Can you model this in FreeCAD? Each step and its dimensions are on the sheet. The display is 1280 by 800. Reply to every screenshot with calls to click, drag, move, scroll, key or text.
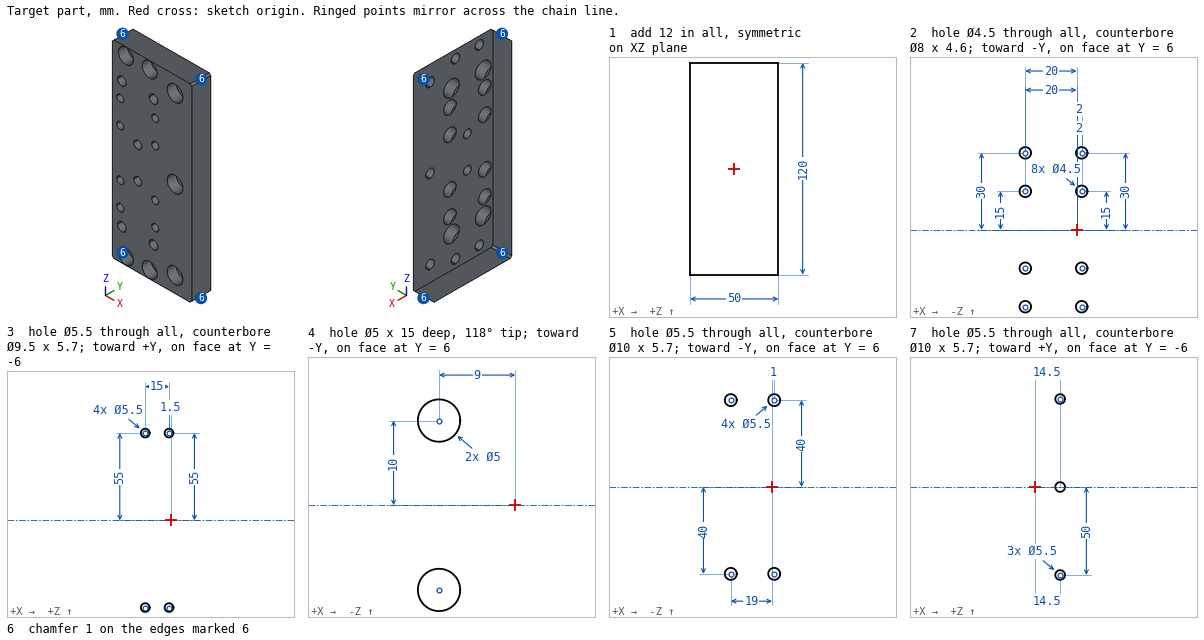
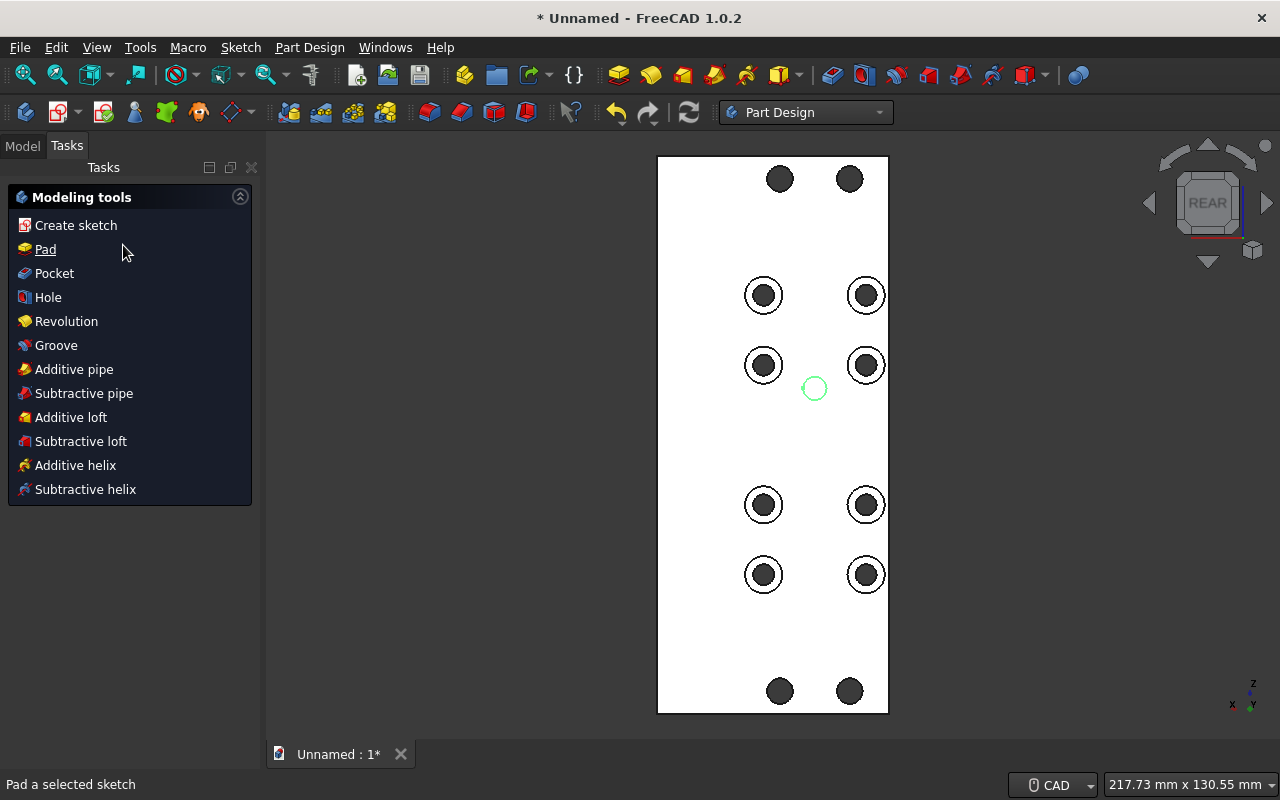
click(866, 76)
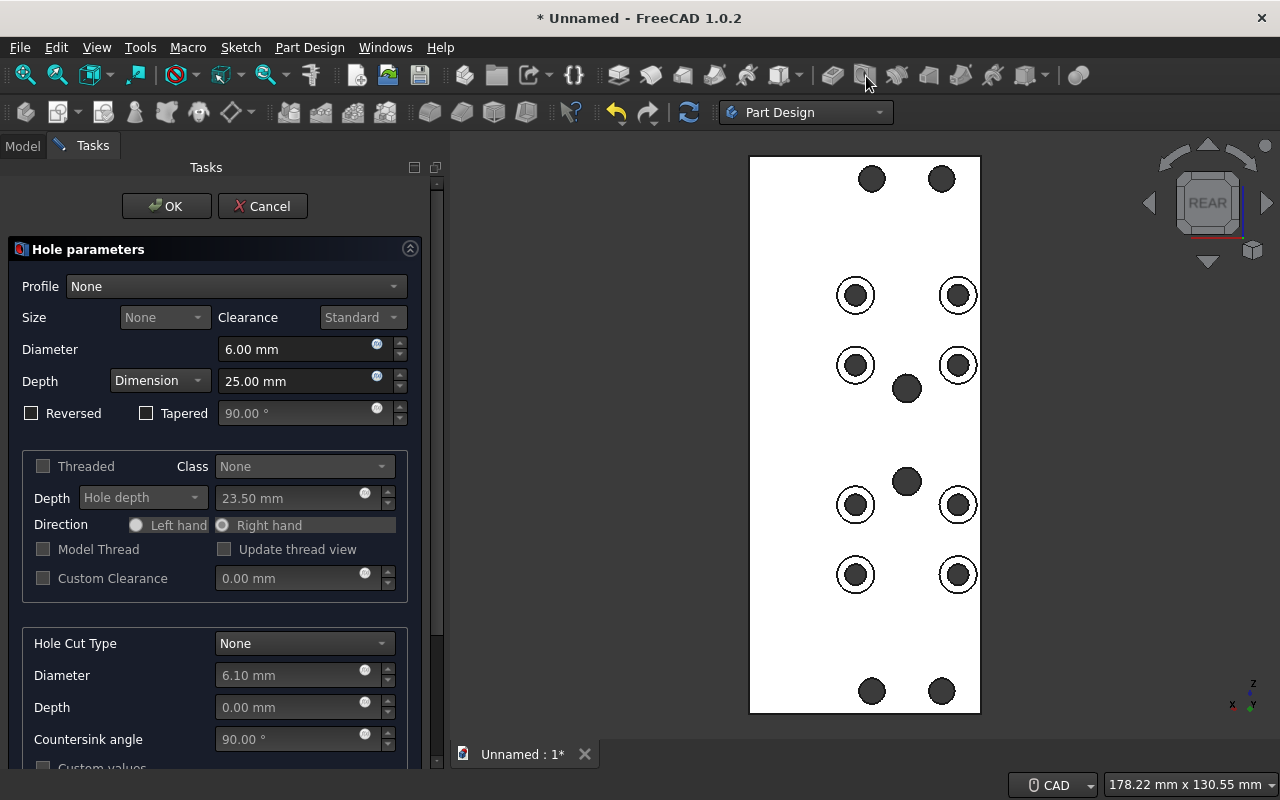
triple_click(305, 349)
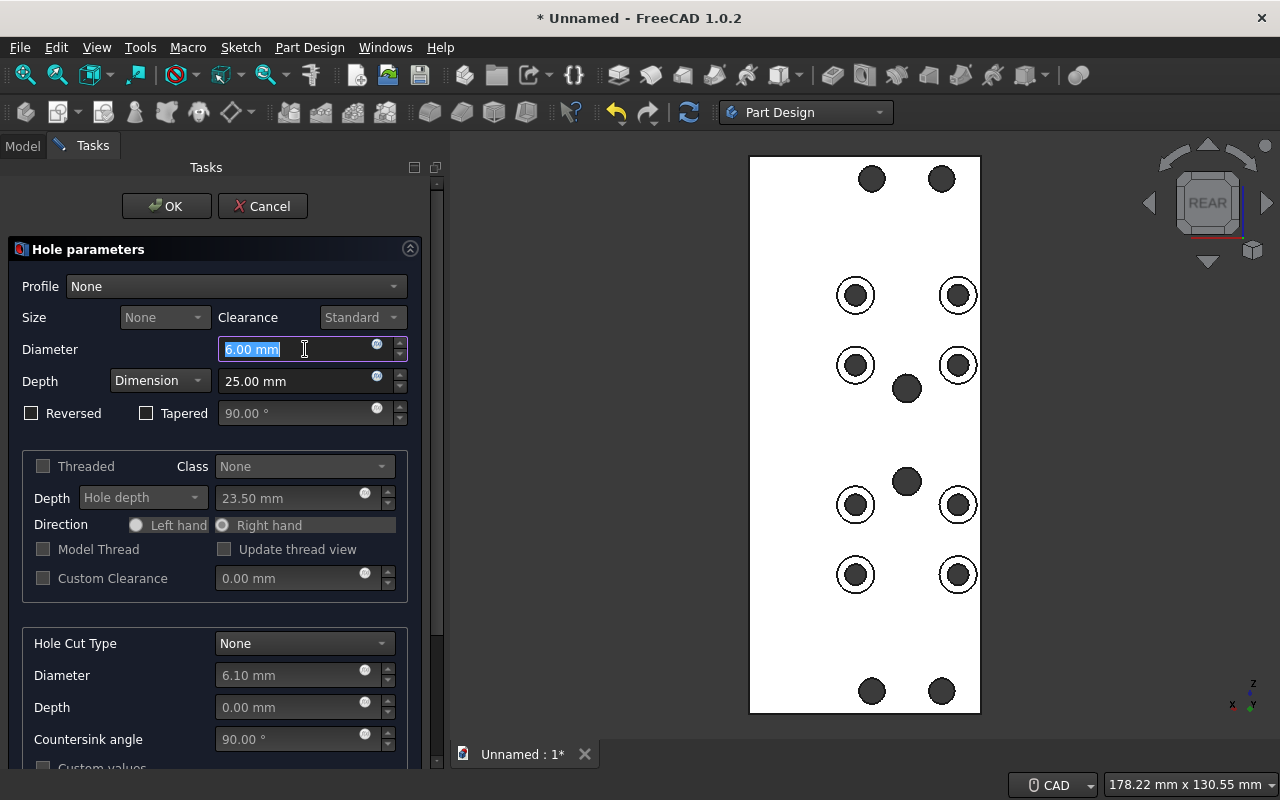
text(5)
key(Tab)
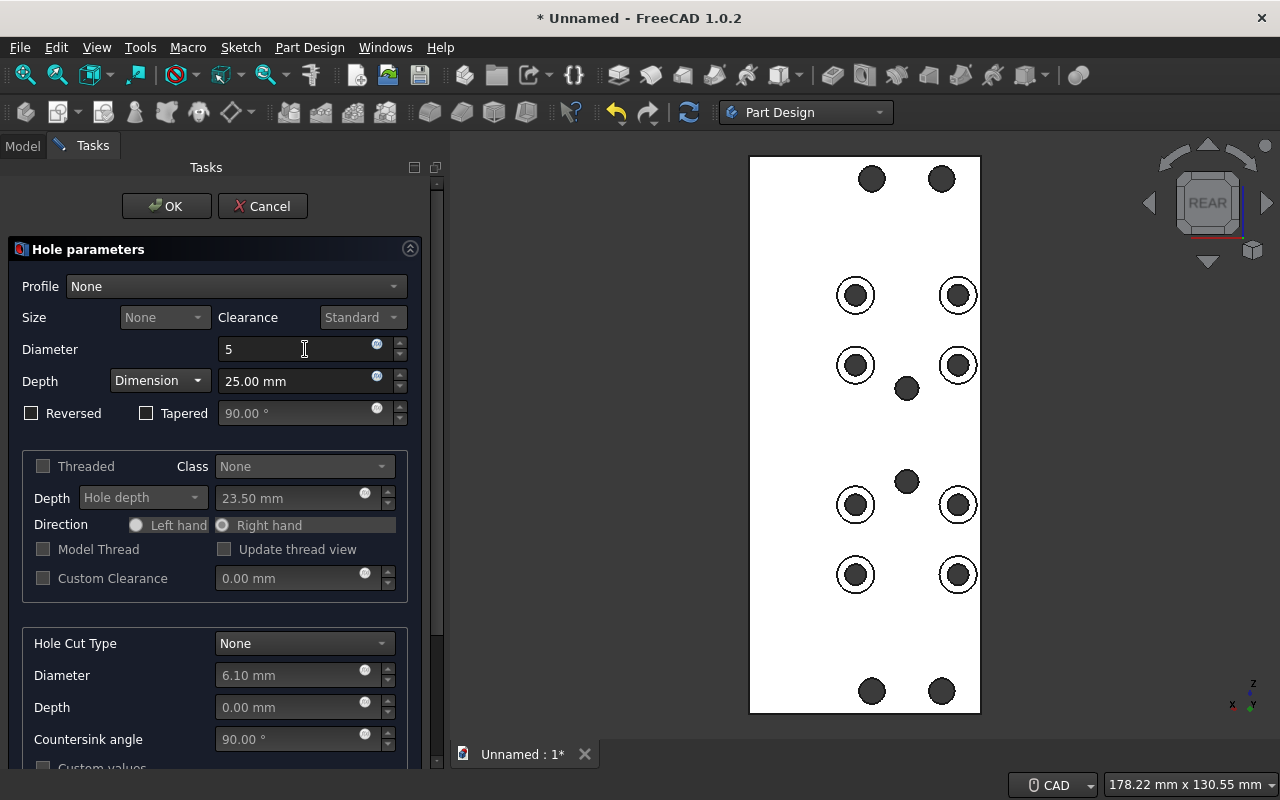
triple_click(305, 381)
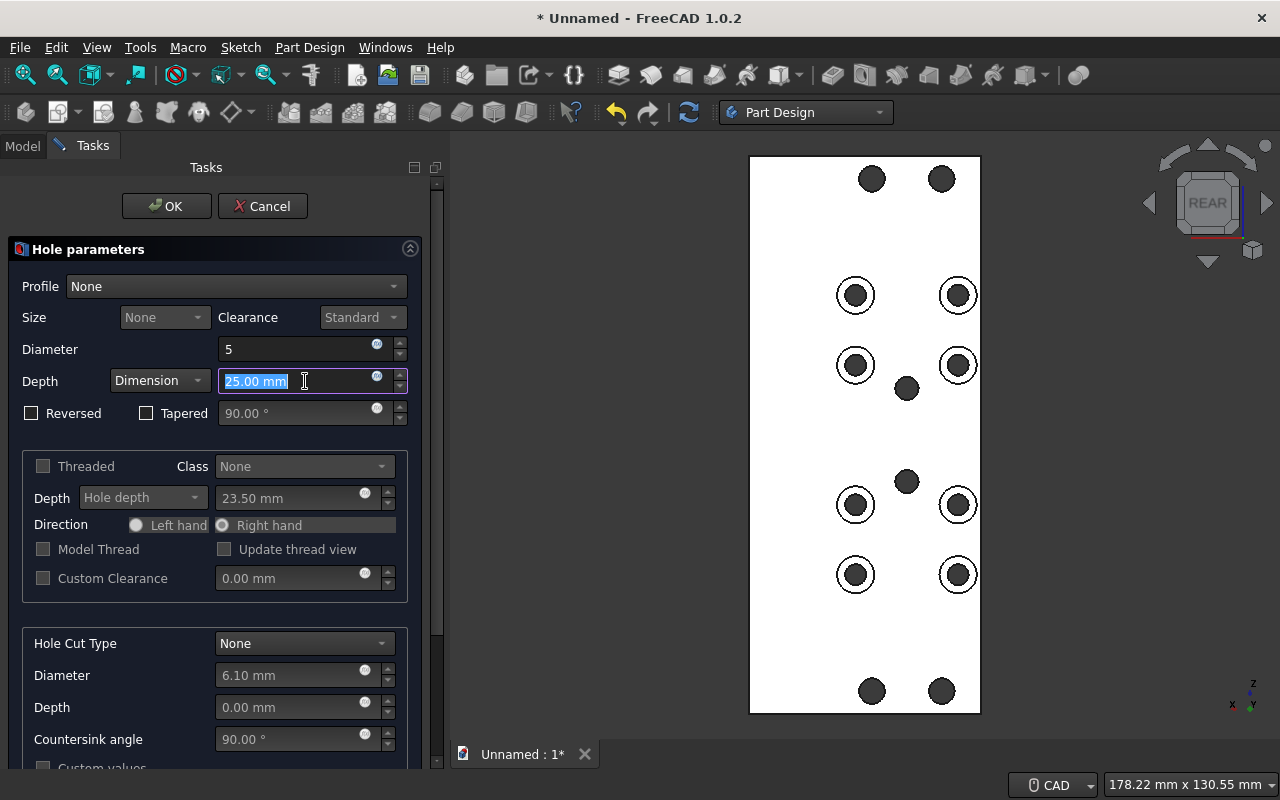
text(15)
key(Tab)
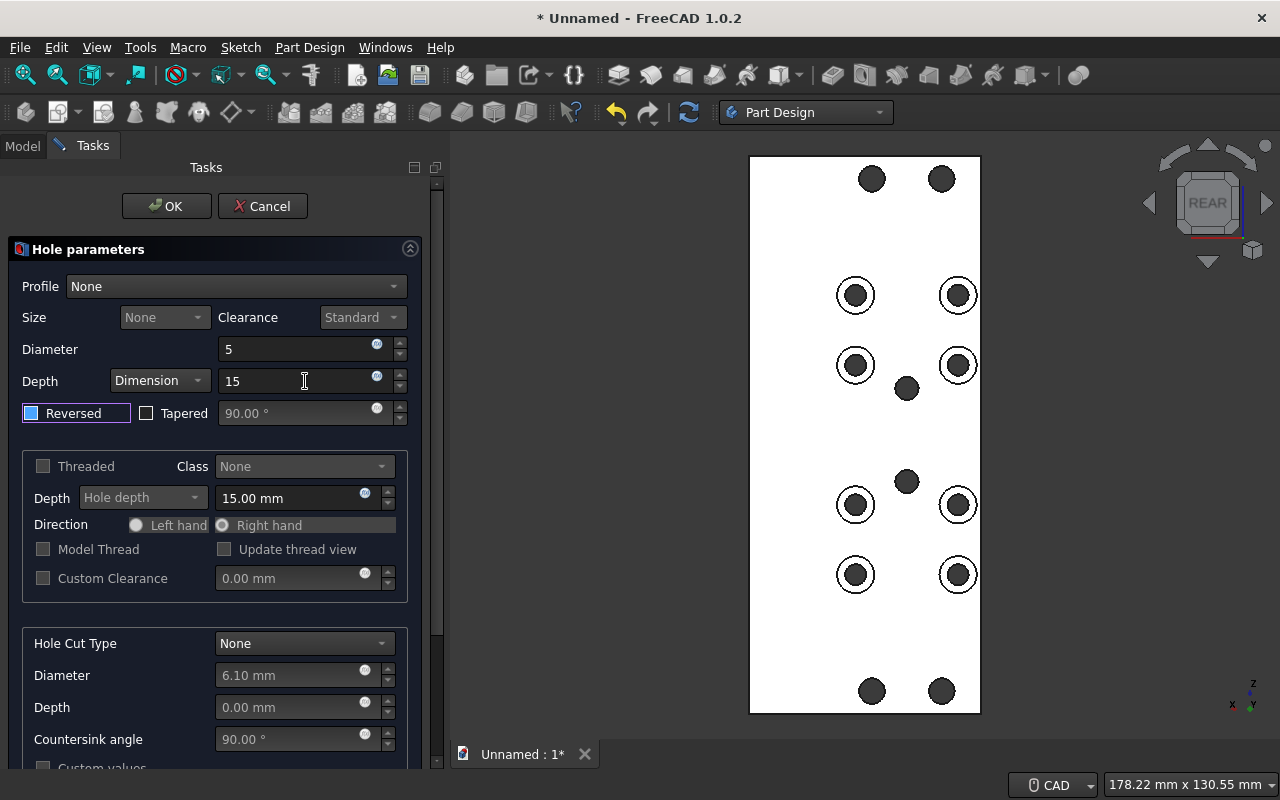
click(167, 206)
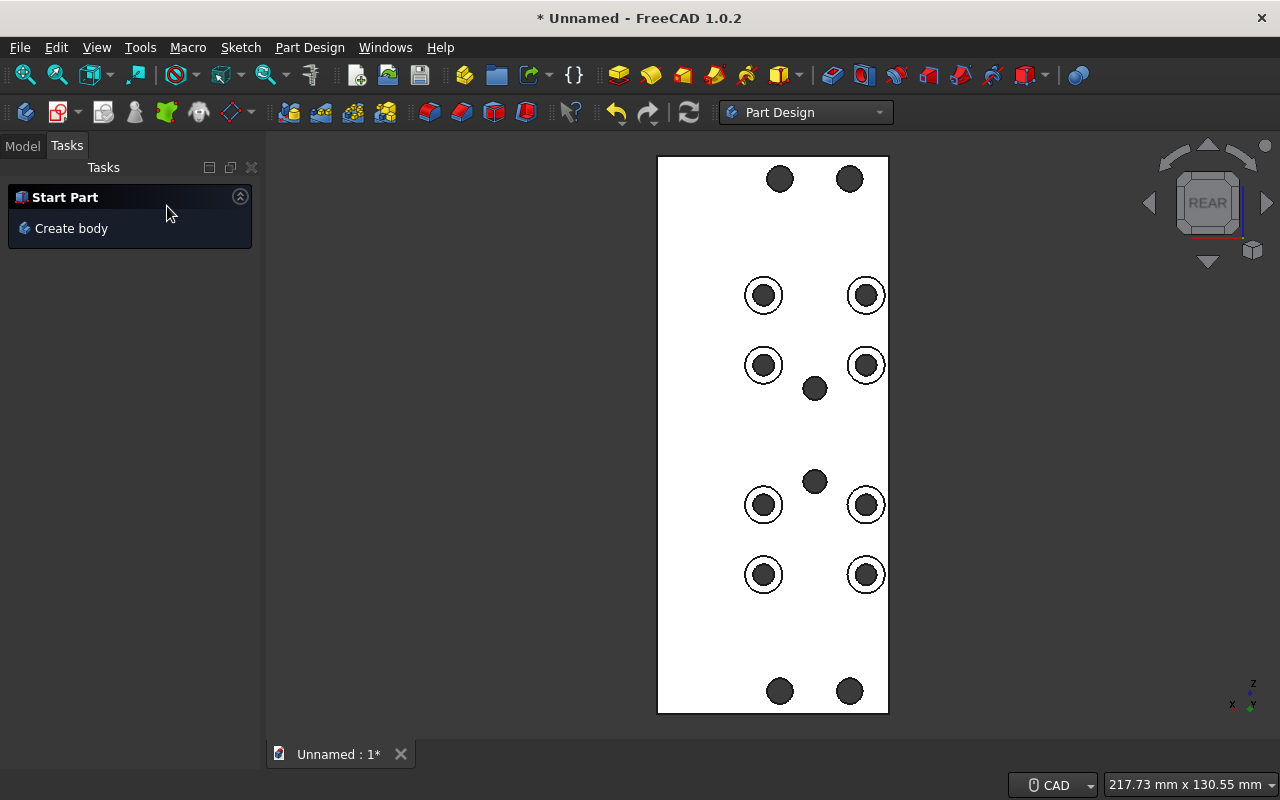
click(740, 434)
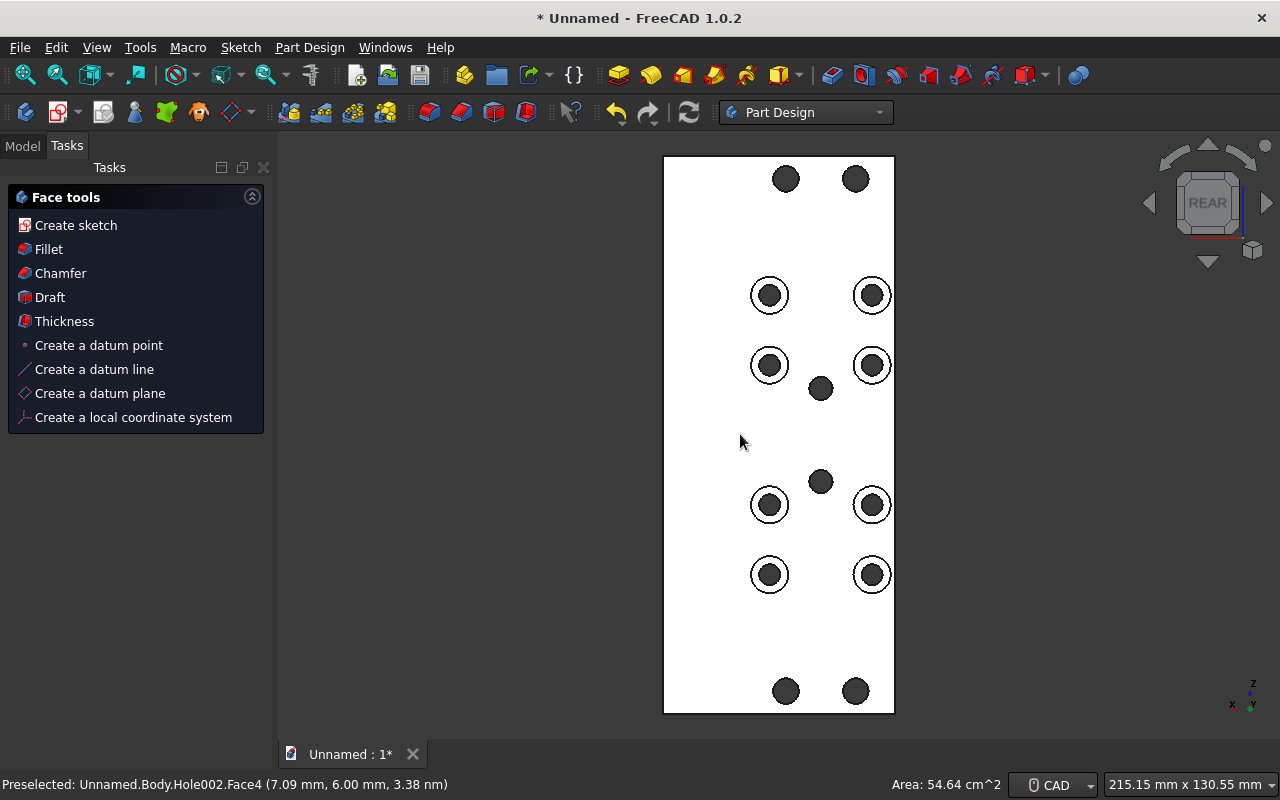
click(58, 112)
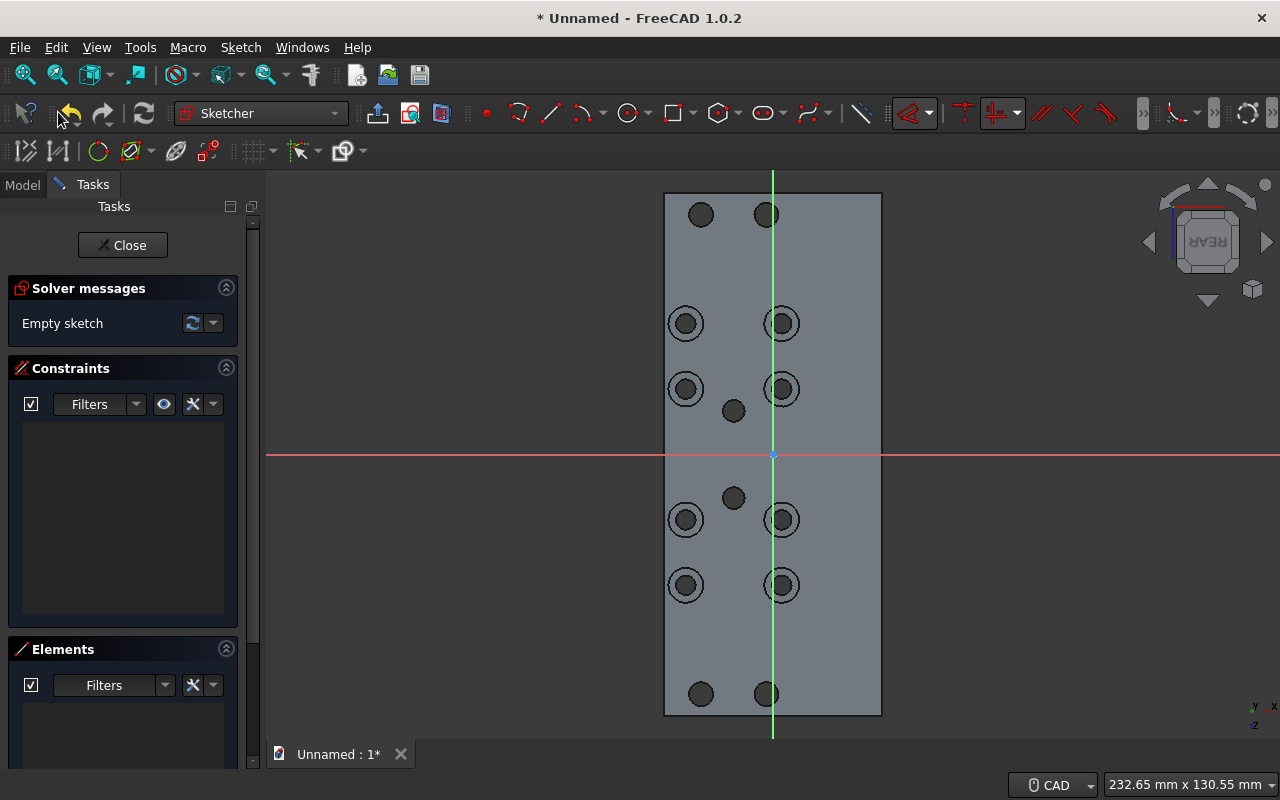
click(628, 114)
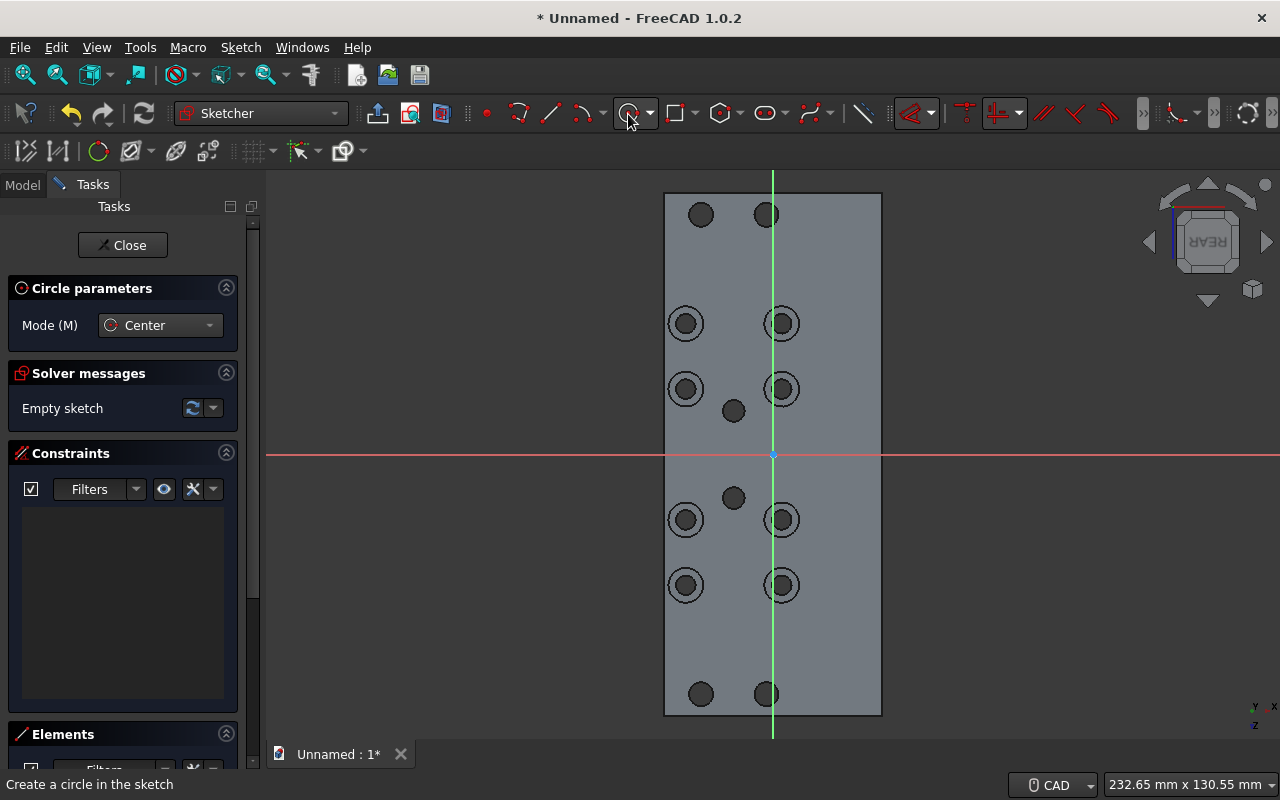
scroll(777, 280, up, 7)